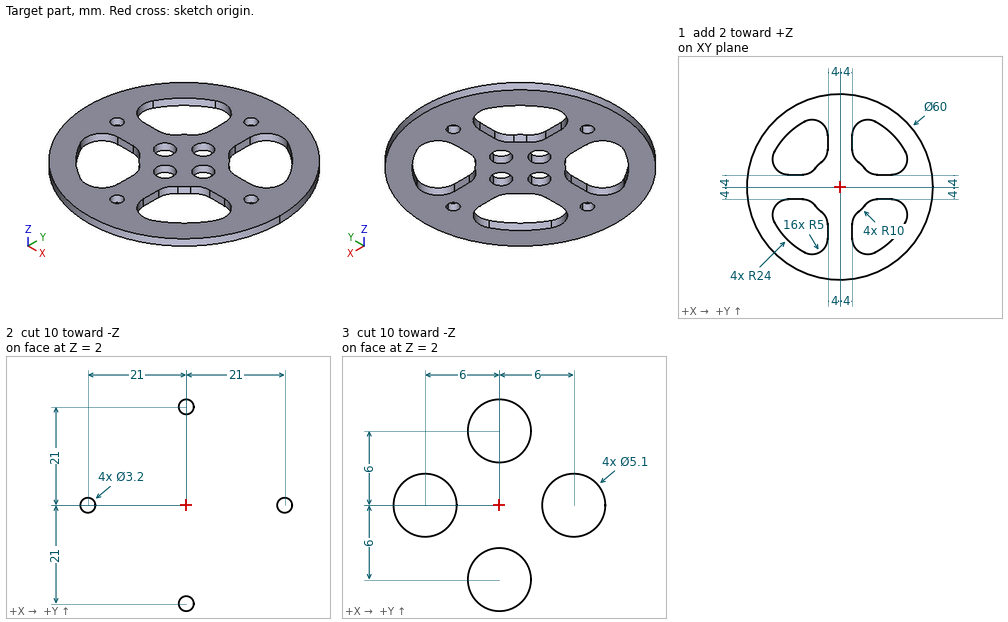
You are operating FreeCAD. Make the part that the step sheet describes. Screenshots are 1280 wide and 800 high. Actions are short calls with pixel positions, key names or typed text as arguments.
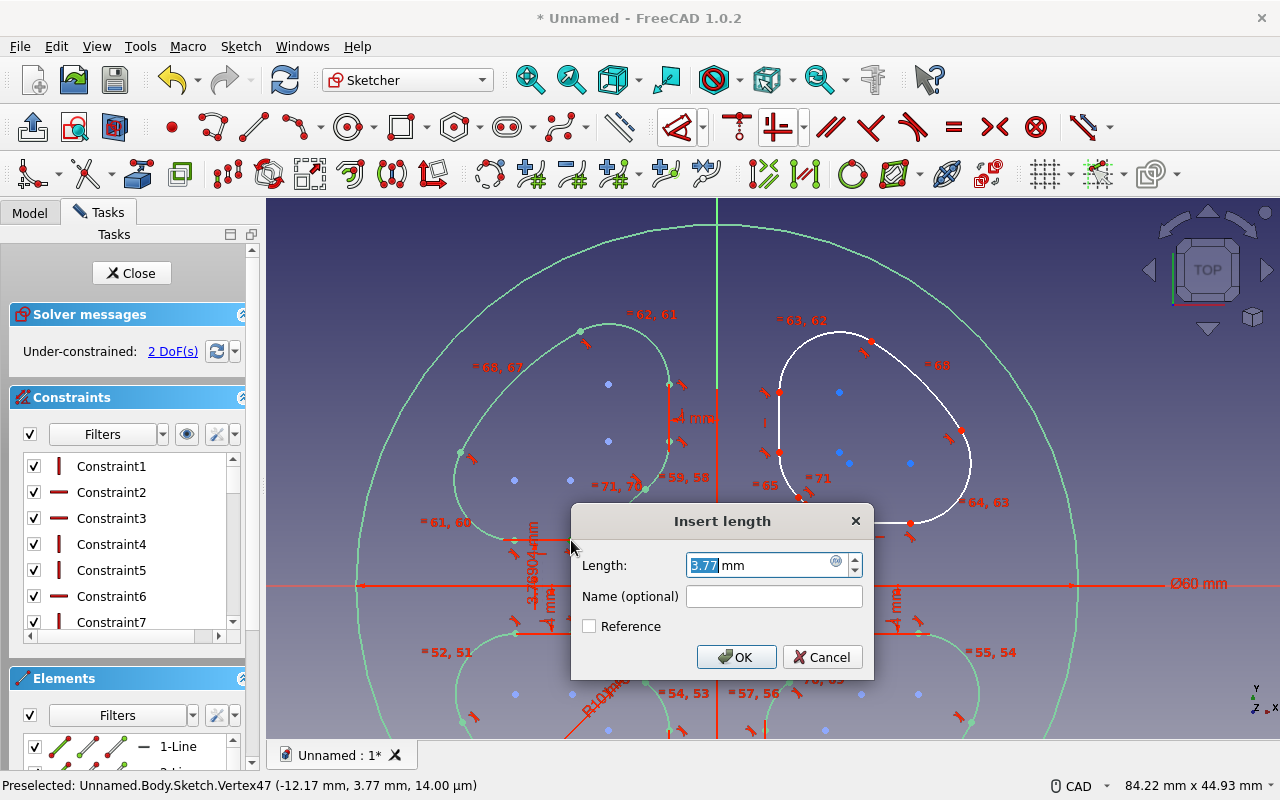
text(4)
key(Return)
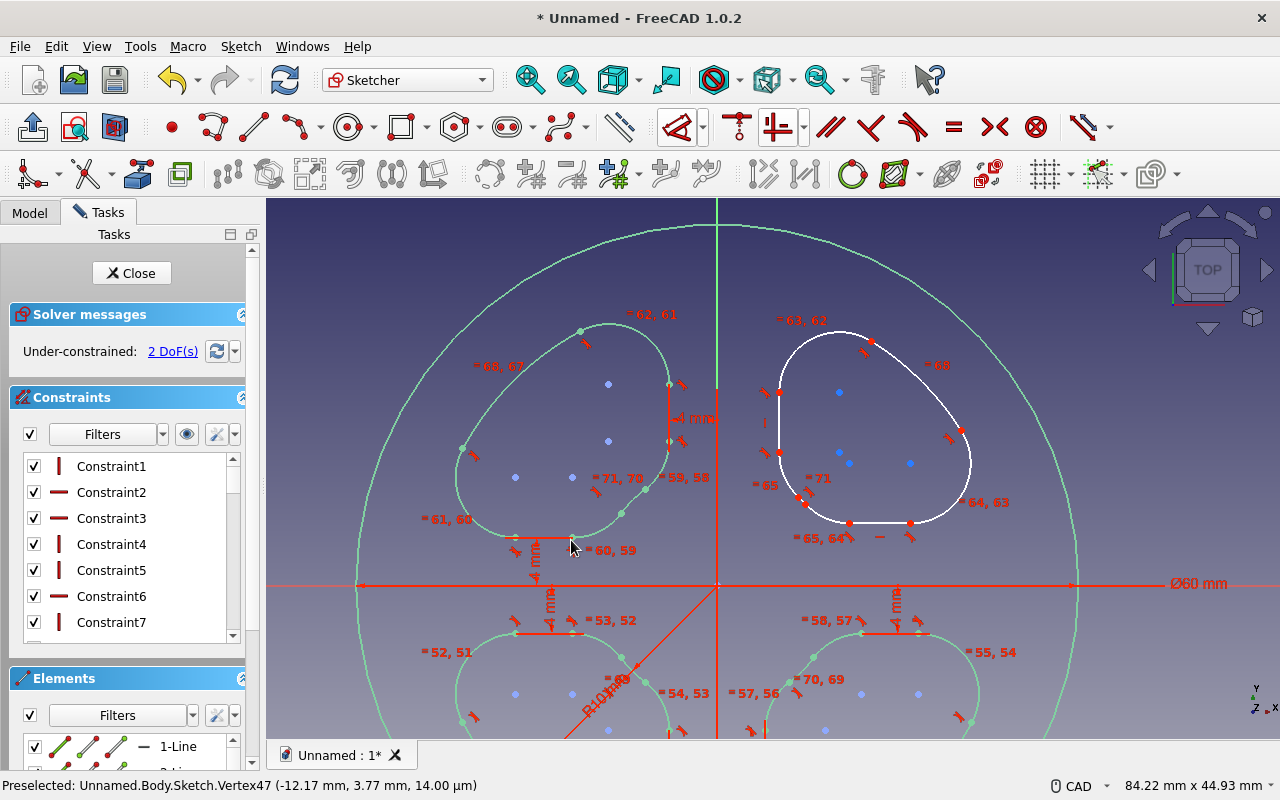
click(779, 453)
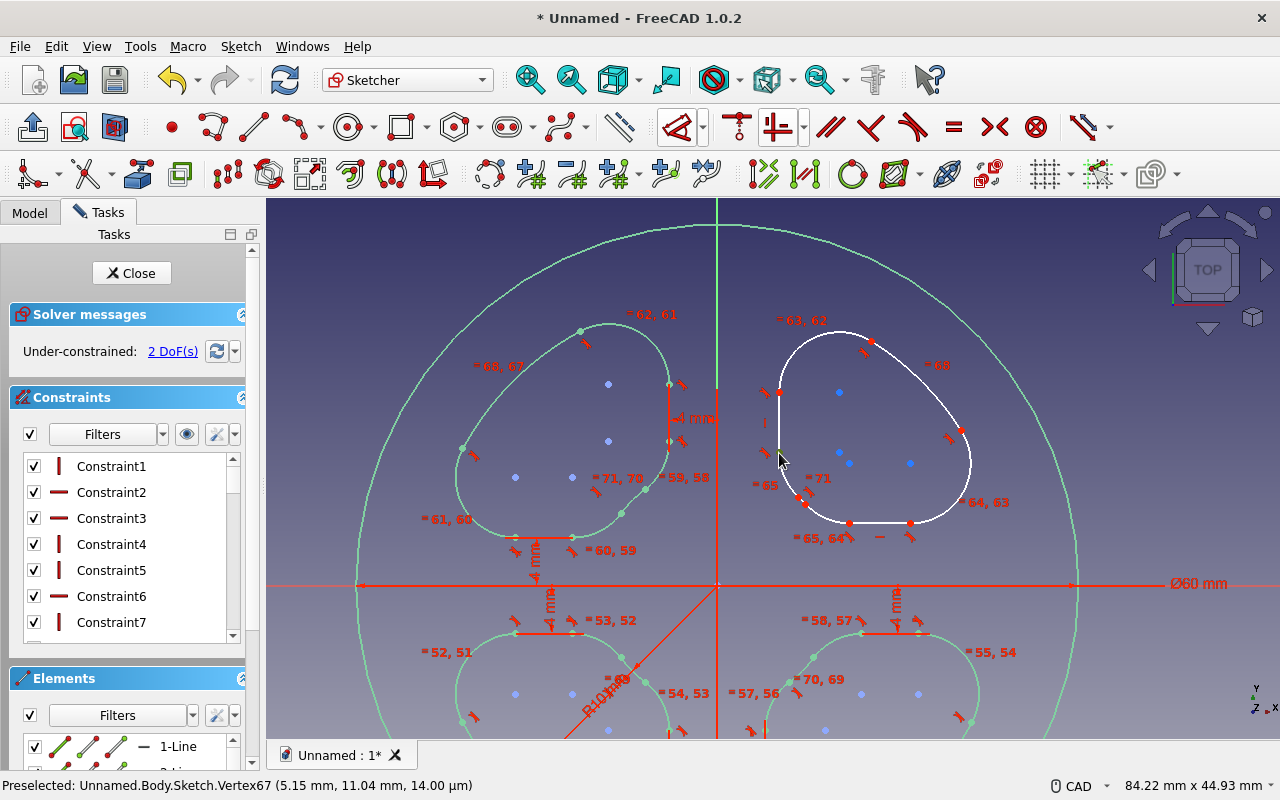
click(702, 128)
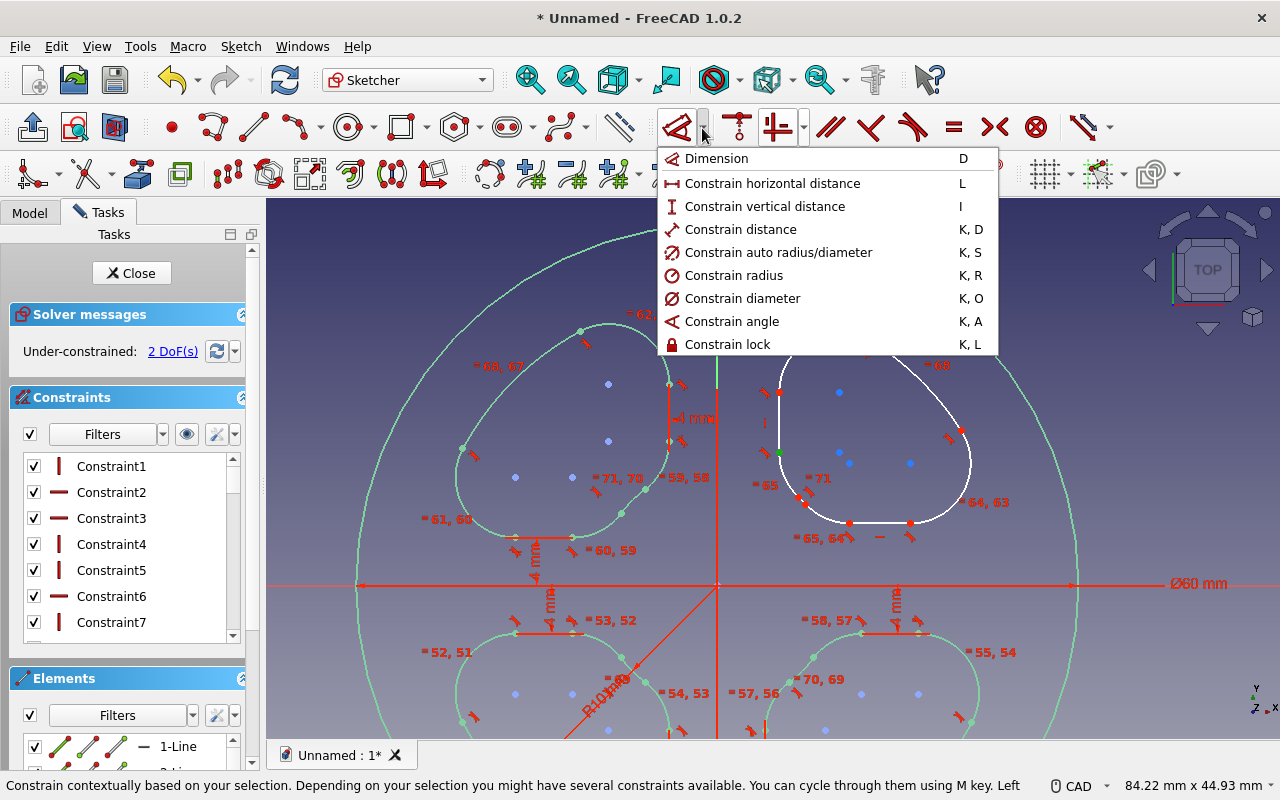
click(828, 184)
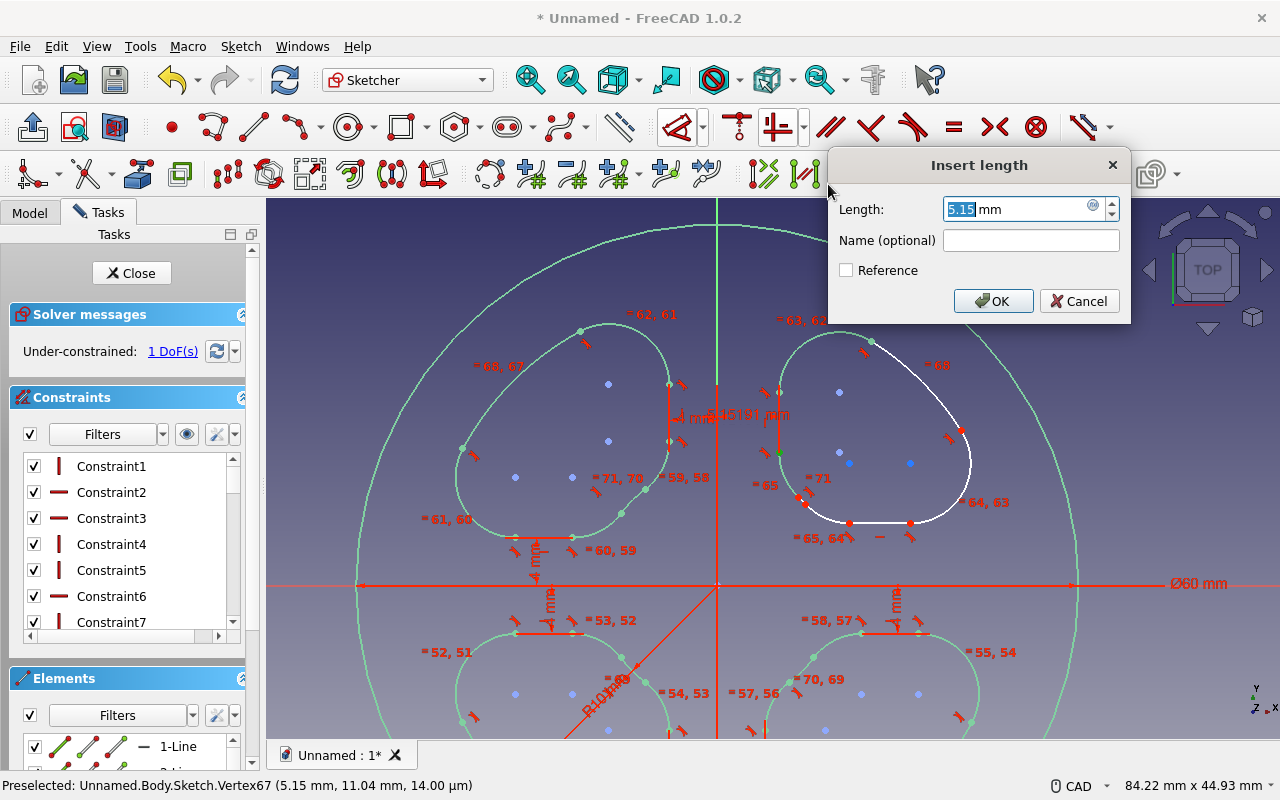
text(4)
key(Return)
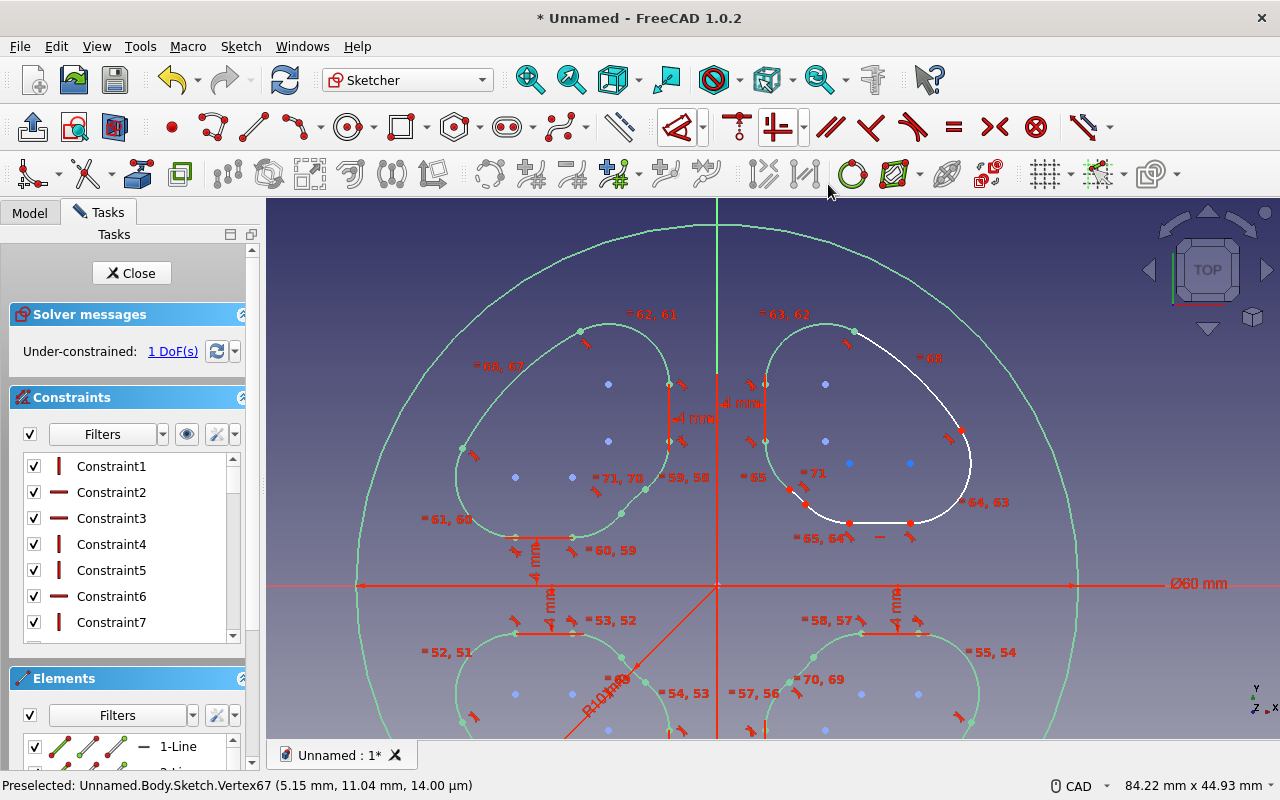
click(910, 523)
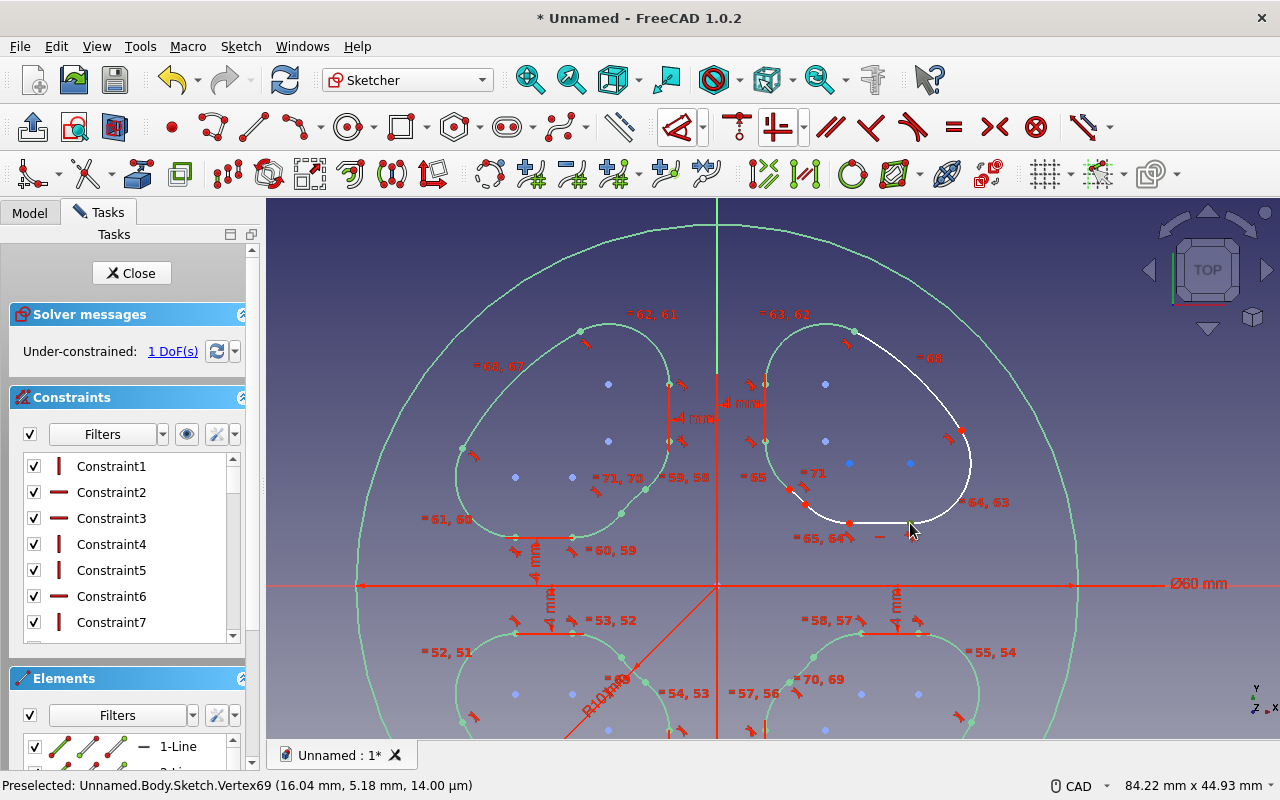
key(i)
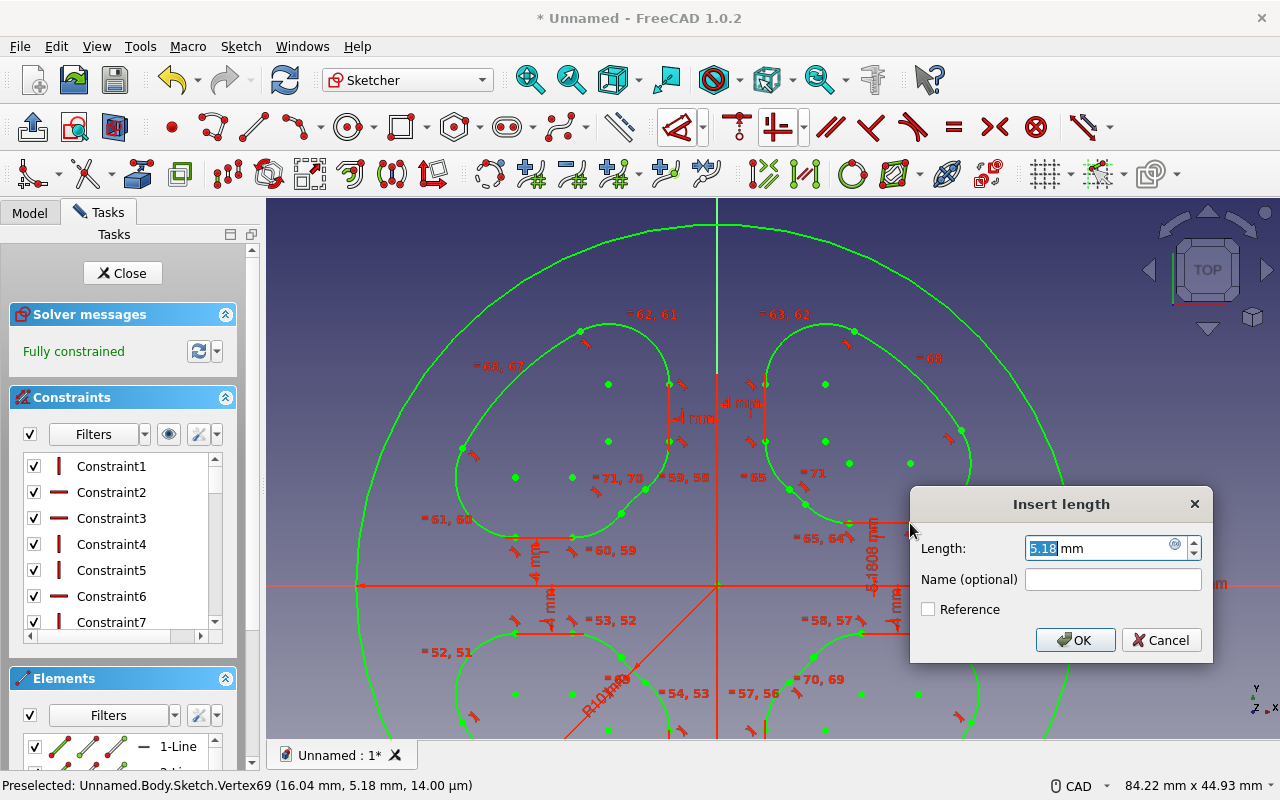
text(4)
key(Return)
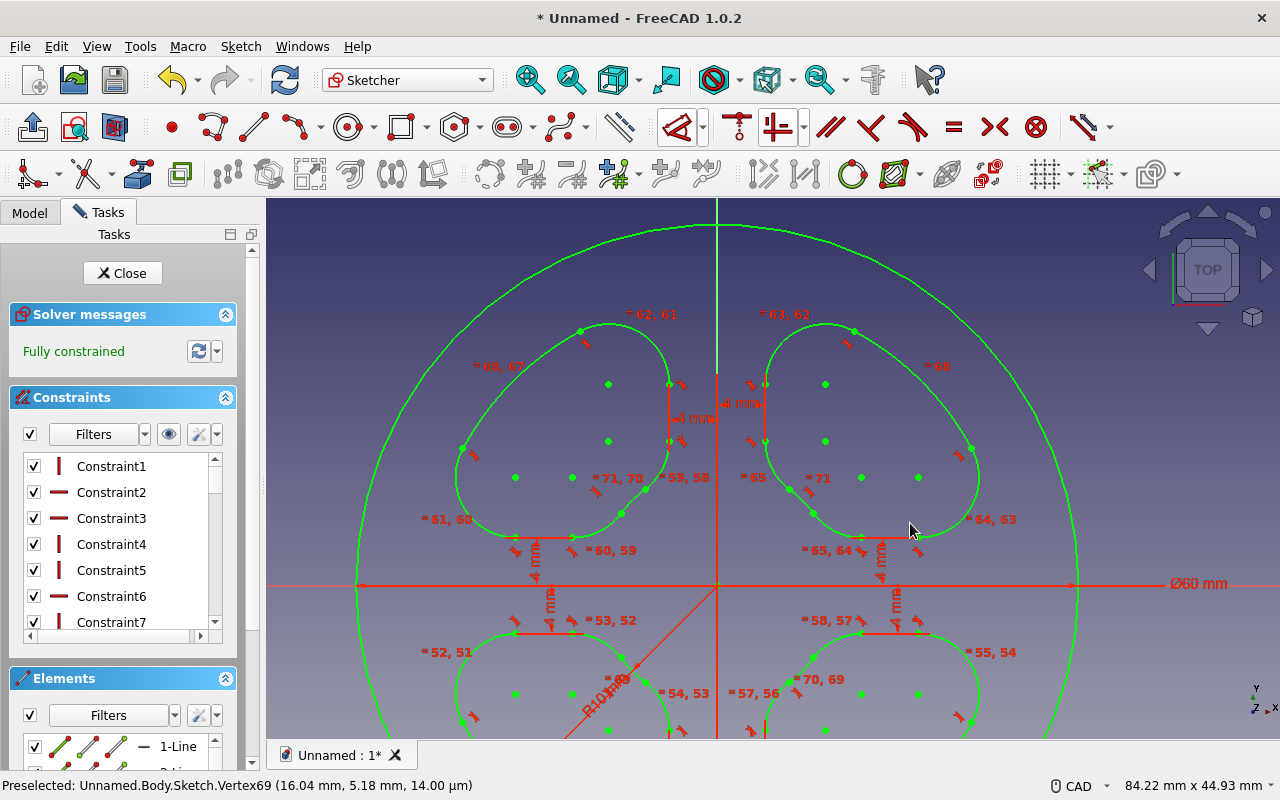
click(123, 273)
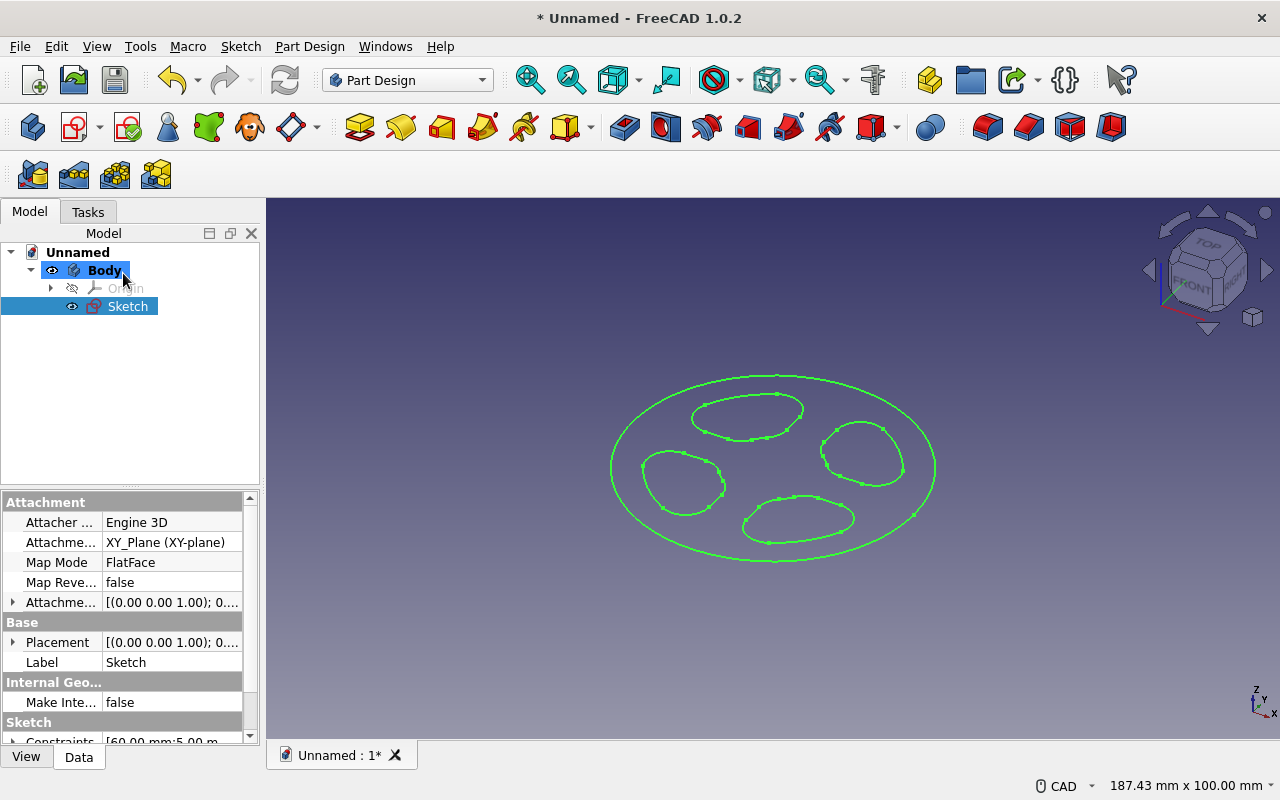
click(360, 128)